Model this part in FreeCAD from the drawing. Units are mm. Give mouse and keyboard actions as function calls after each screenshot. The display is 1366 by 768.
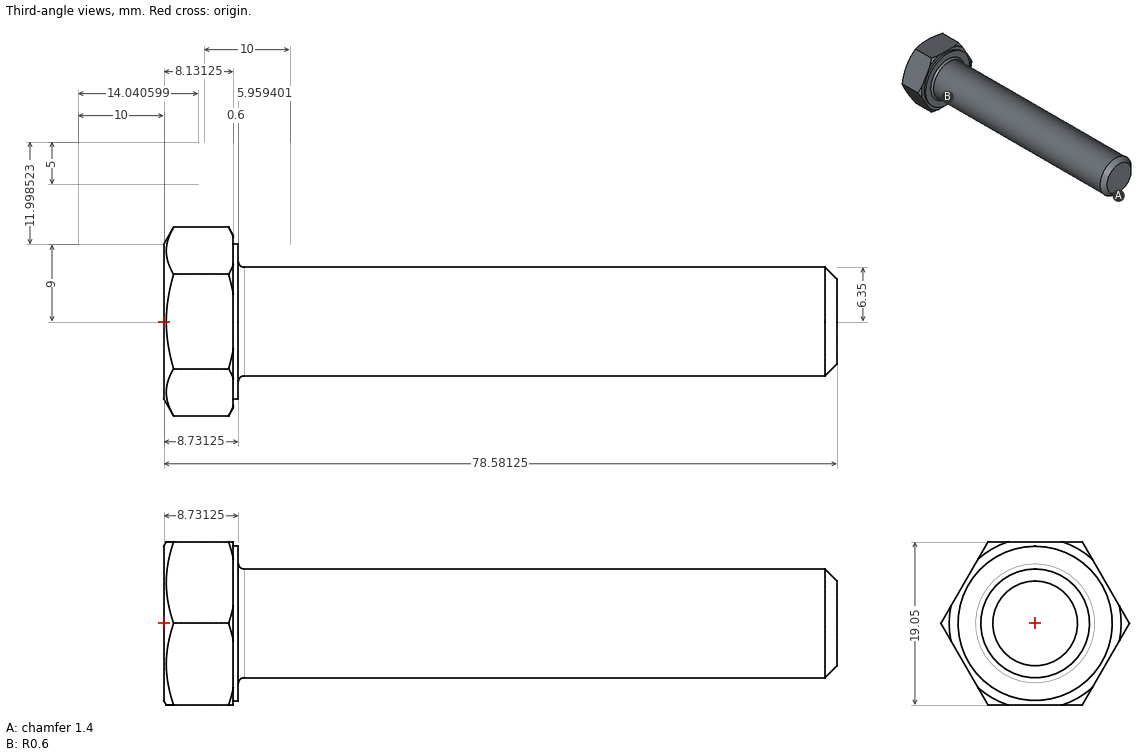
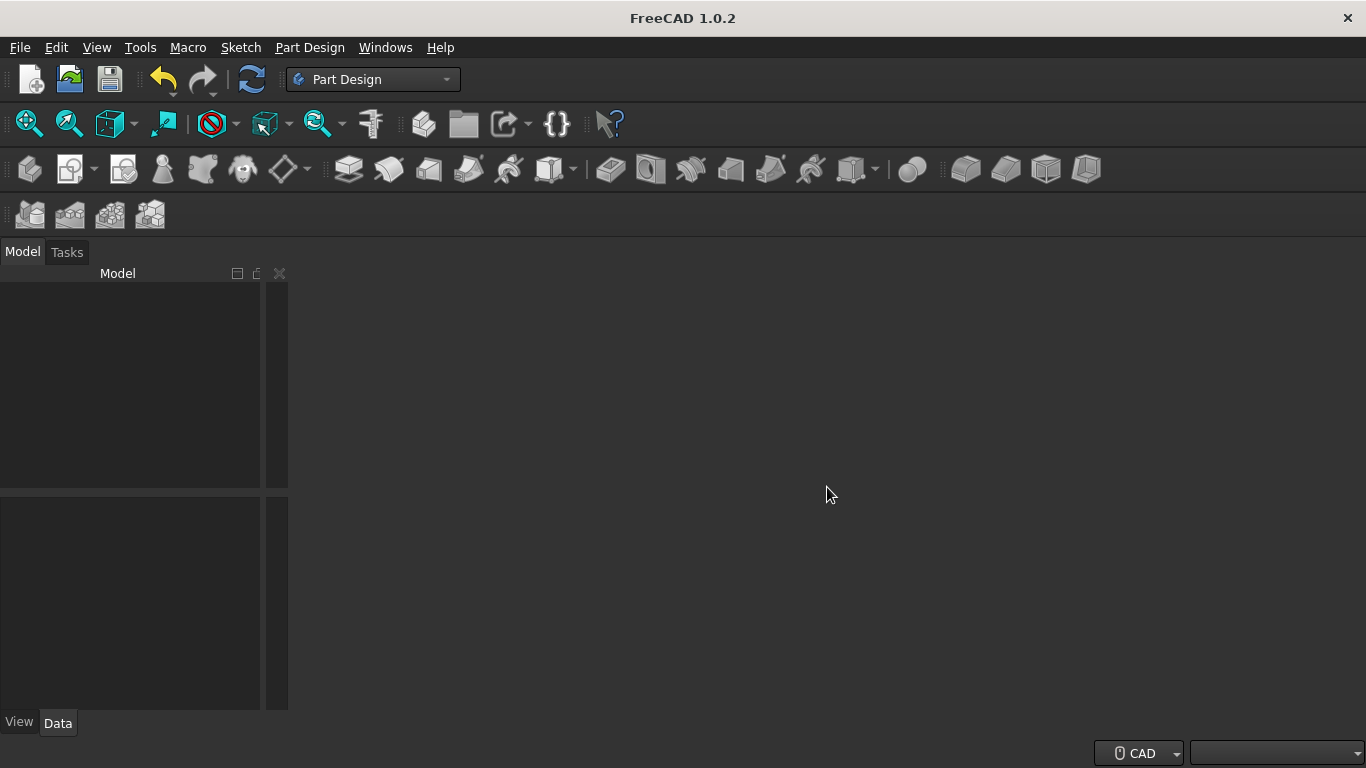
click(30, 80)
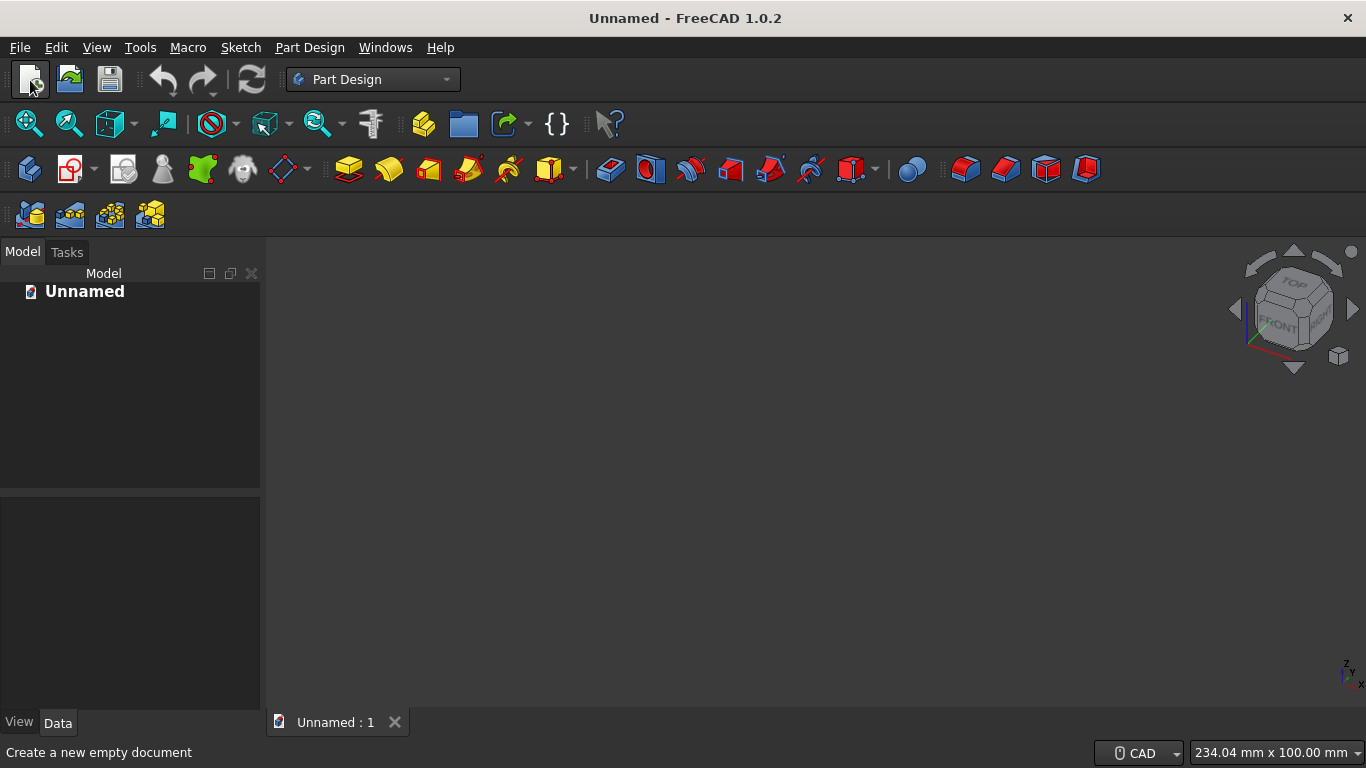
click(70, 170)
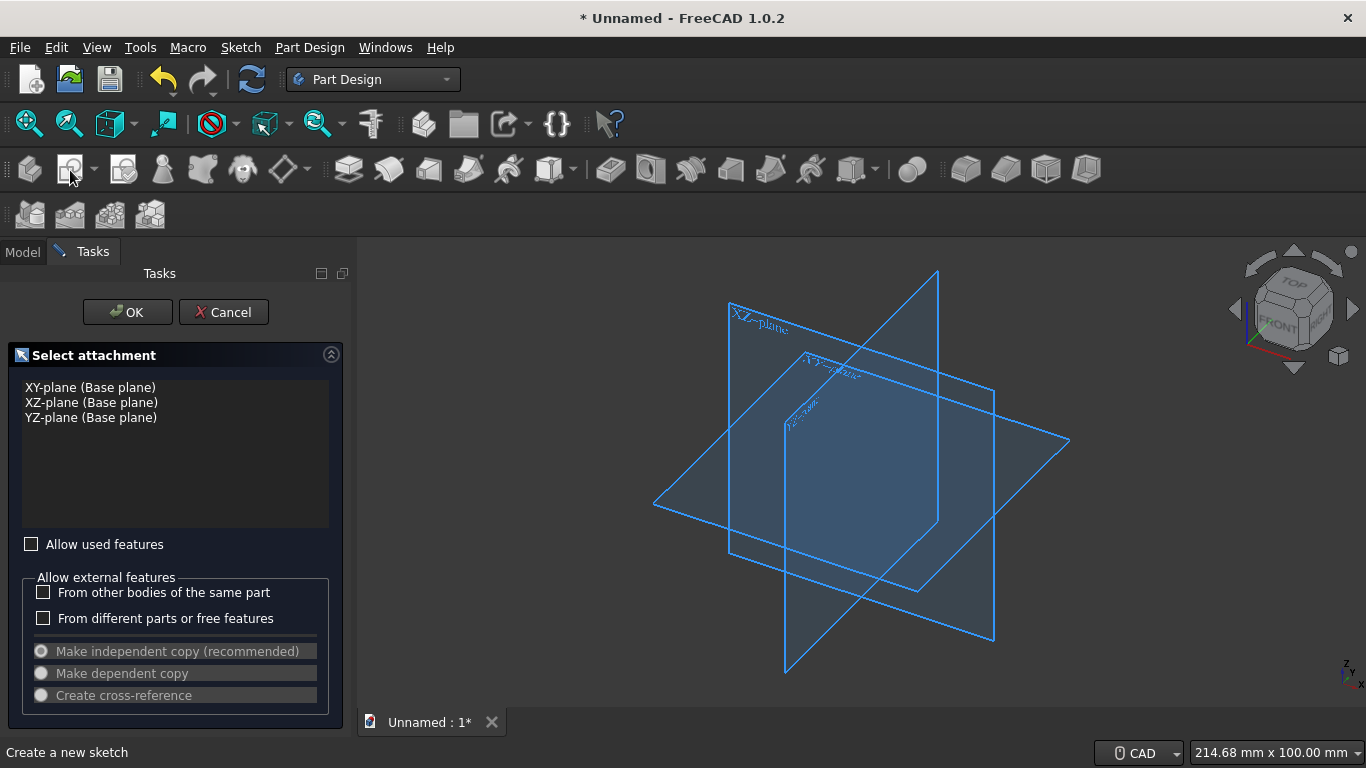
click(82, 418)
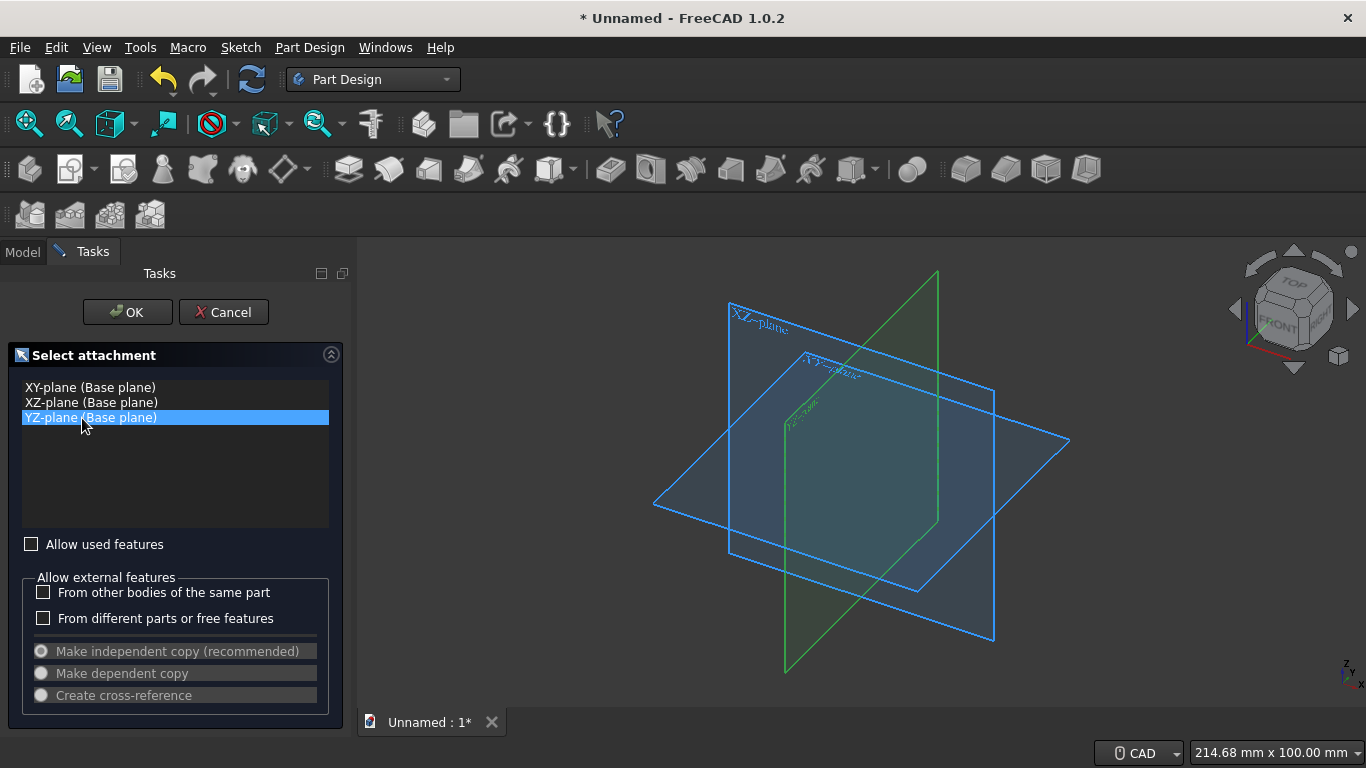
click(128, 312)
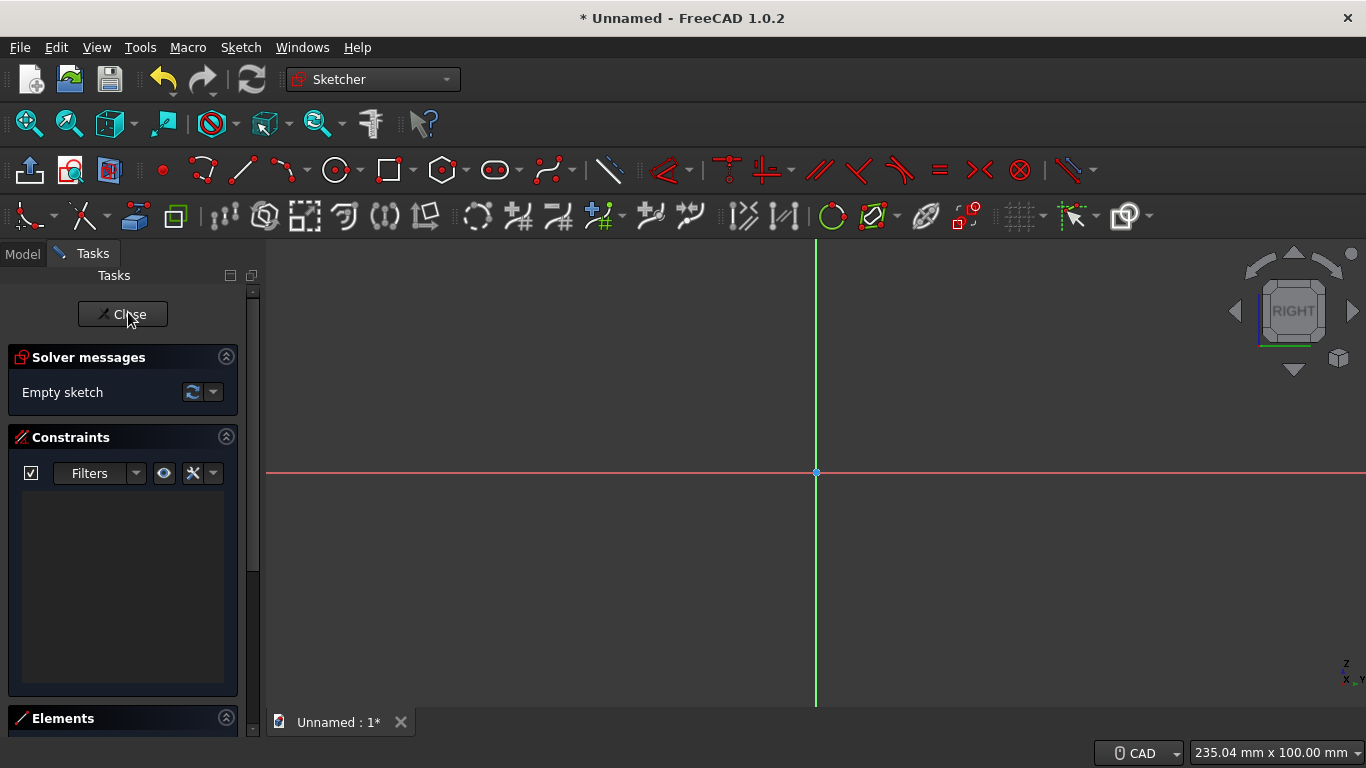
scroll(846, 473, up, 6)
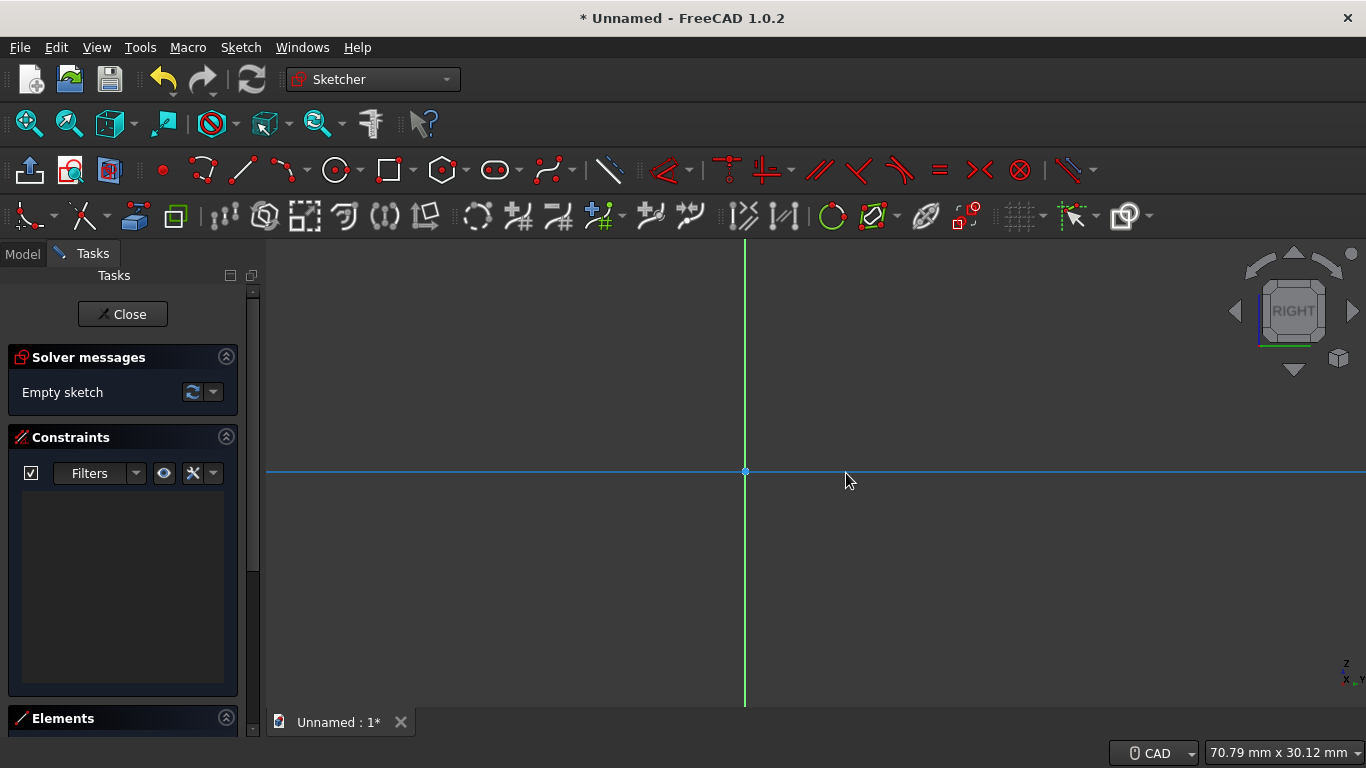
click(442, 170)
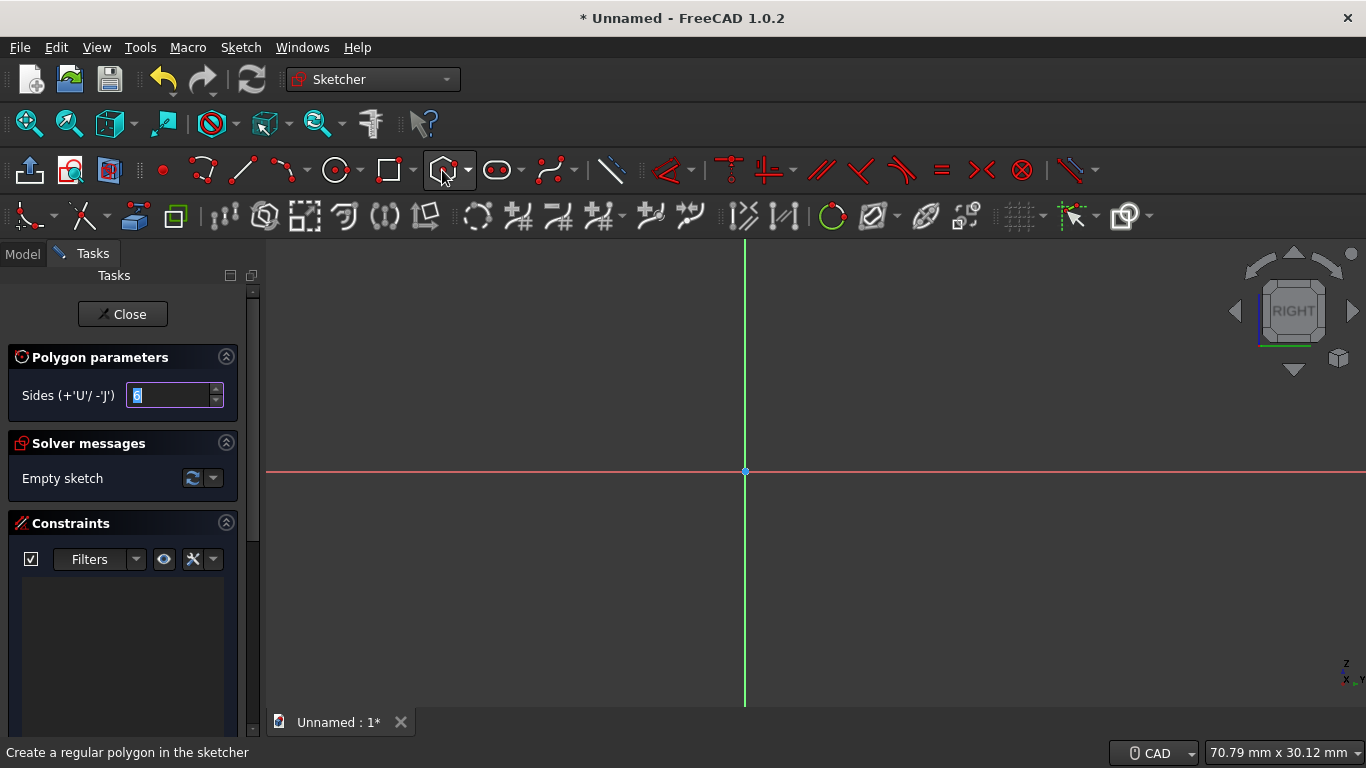
click(745, 472)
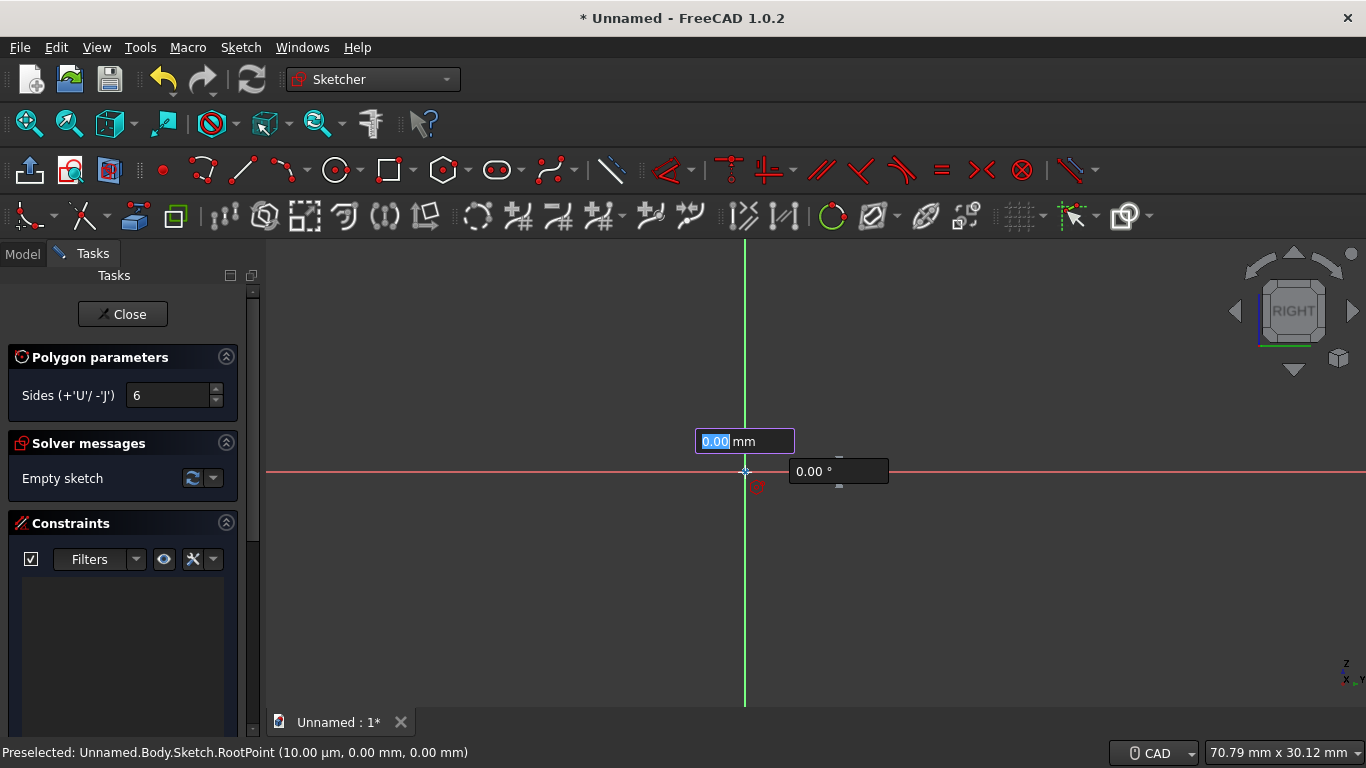
click(916, 472)
key(Escape)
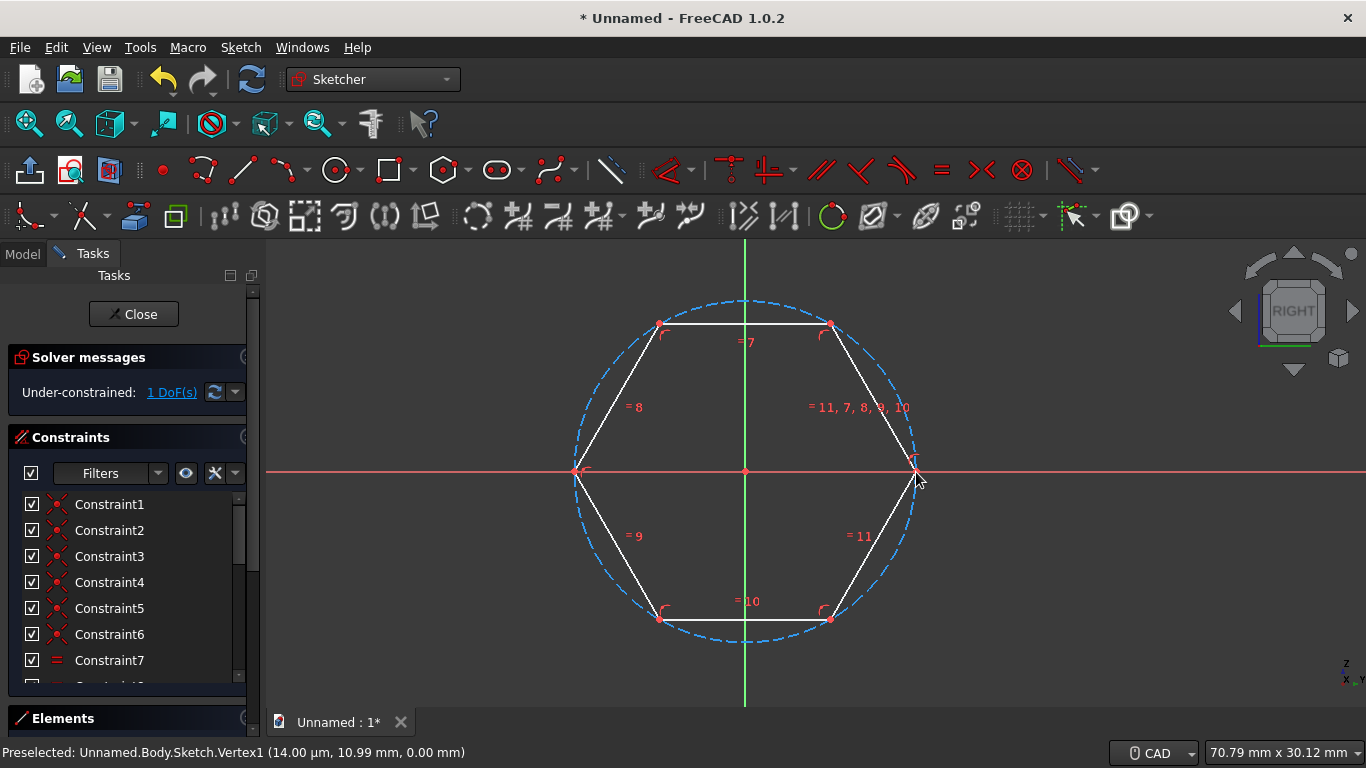
click(666, 170)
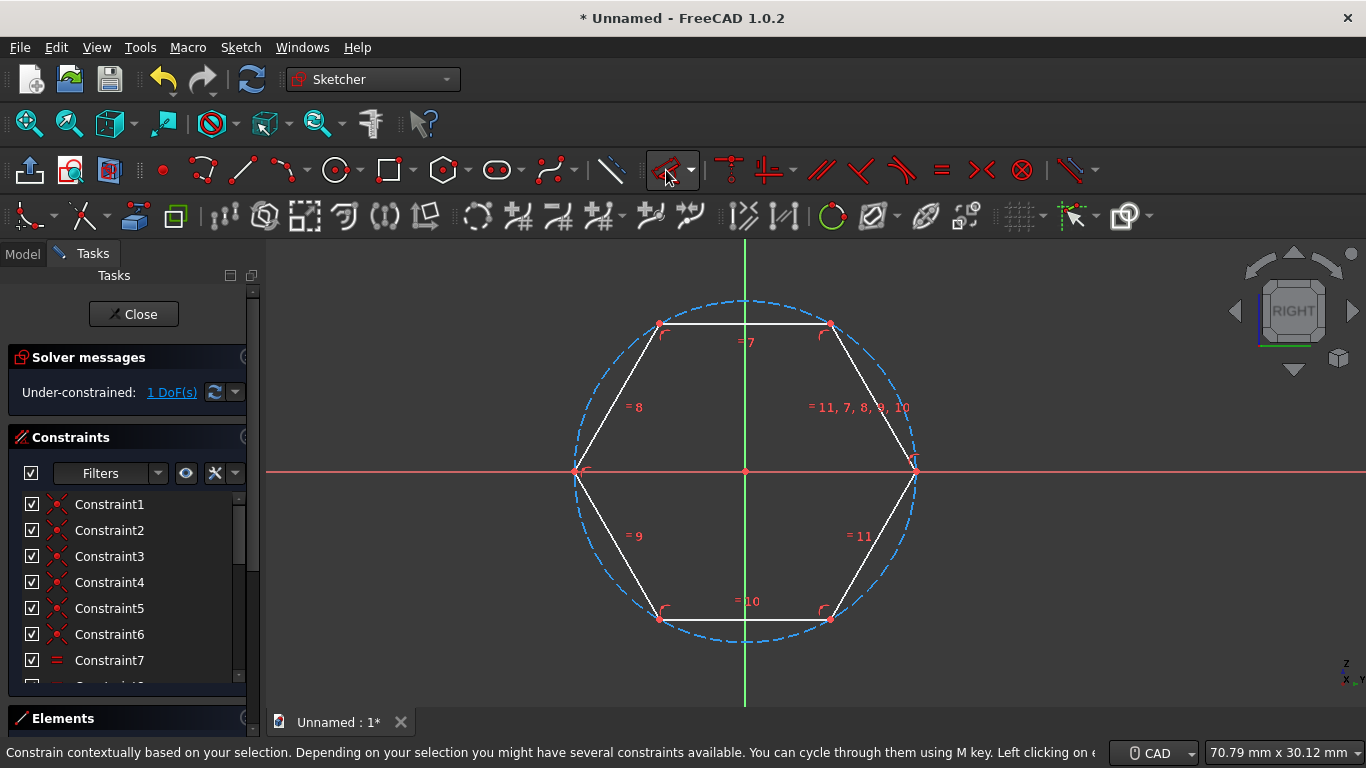
click(660, 620)